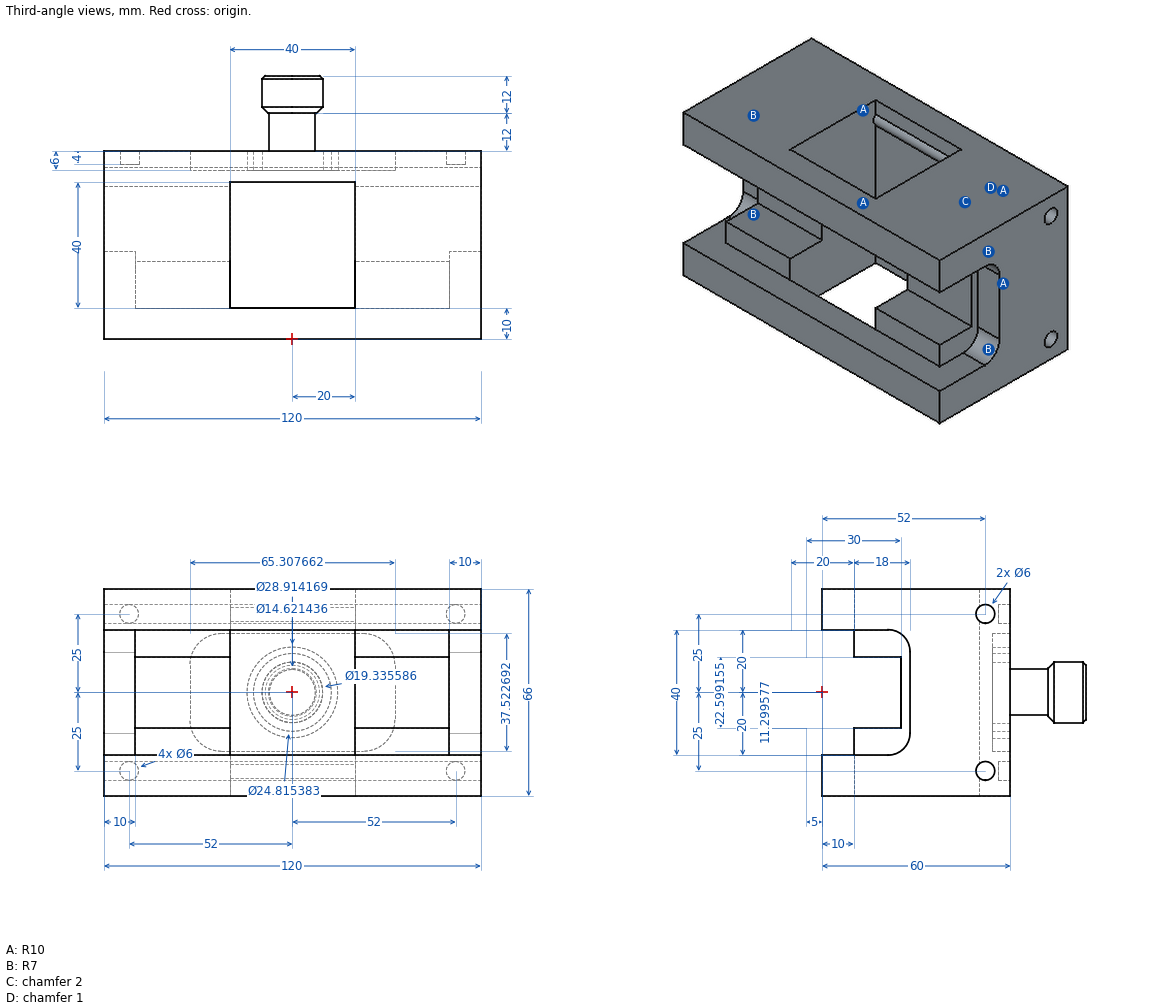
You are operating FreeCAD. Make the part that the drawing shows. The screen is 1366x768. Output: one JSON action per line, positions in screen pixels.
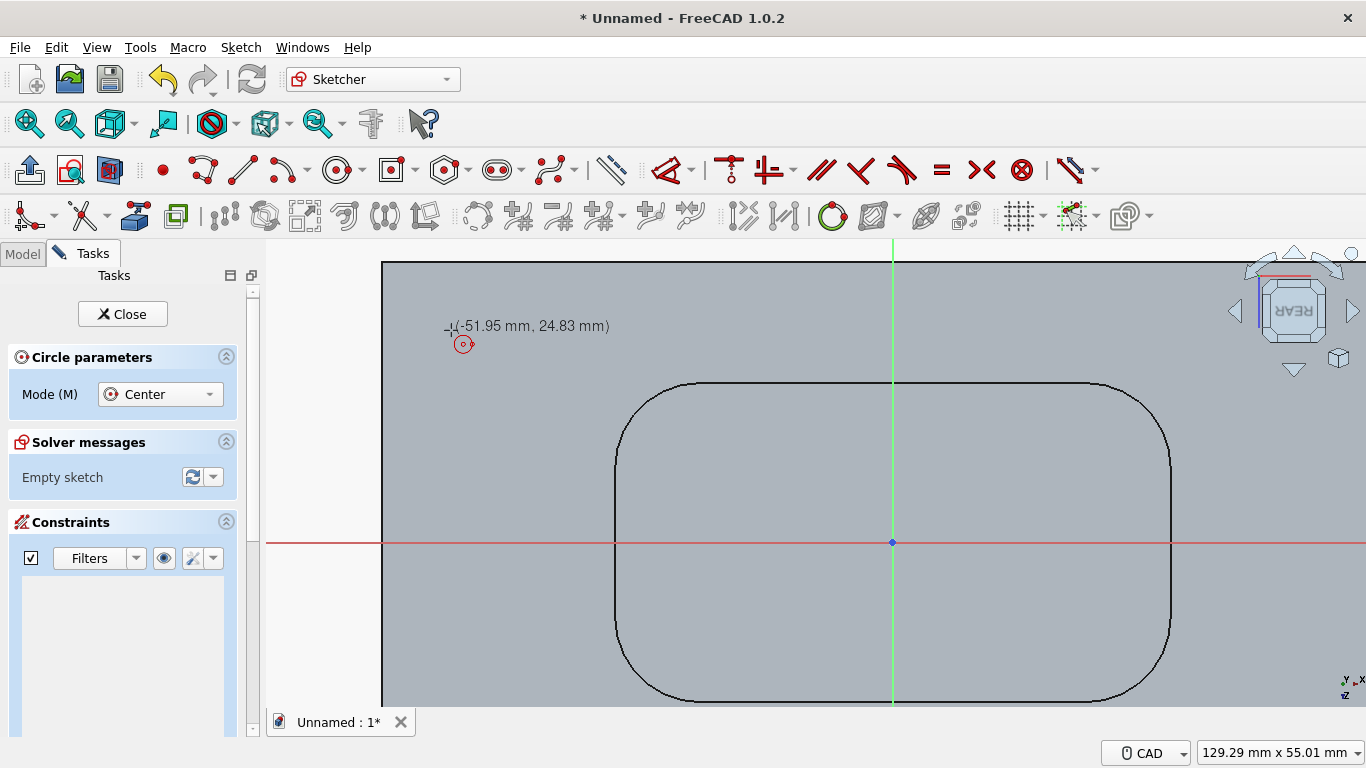
{"action": "left_click", "coordinate": [450, 330]}
{"action": "mouse_move", "coordinate": [469, 312]}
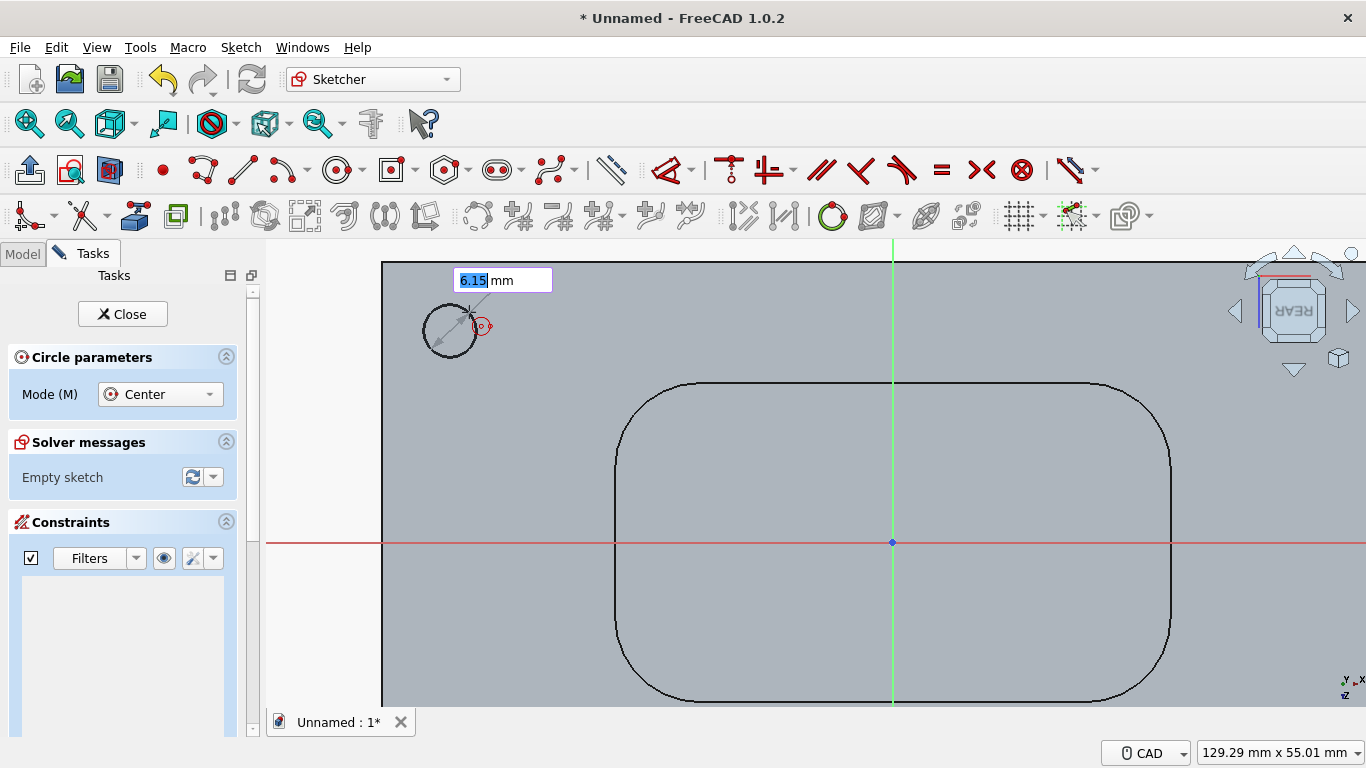
{"action": "type", "text": "6"}
{"action": "key", "text": "Return"}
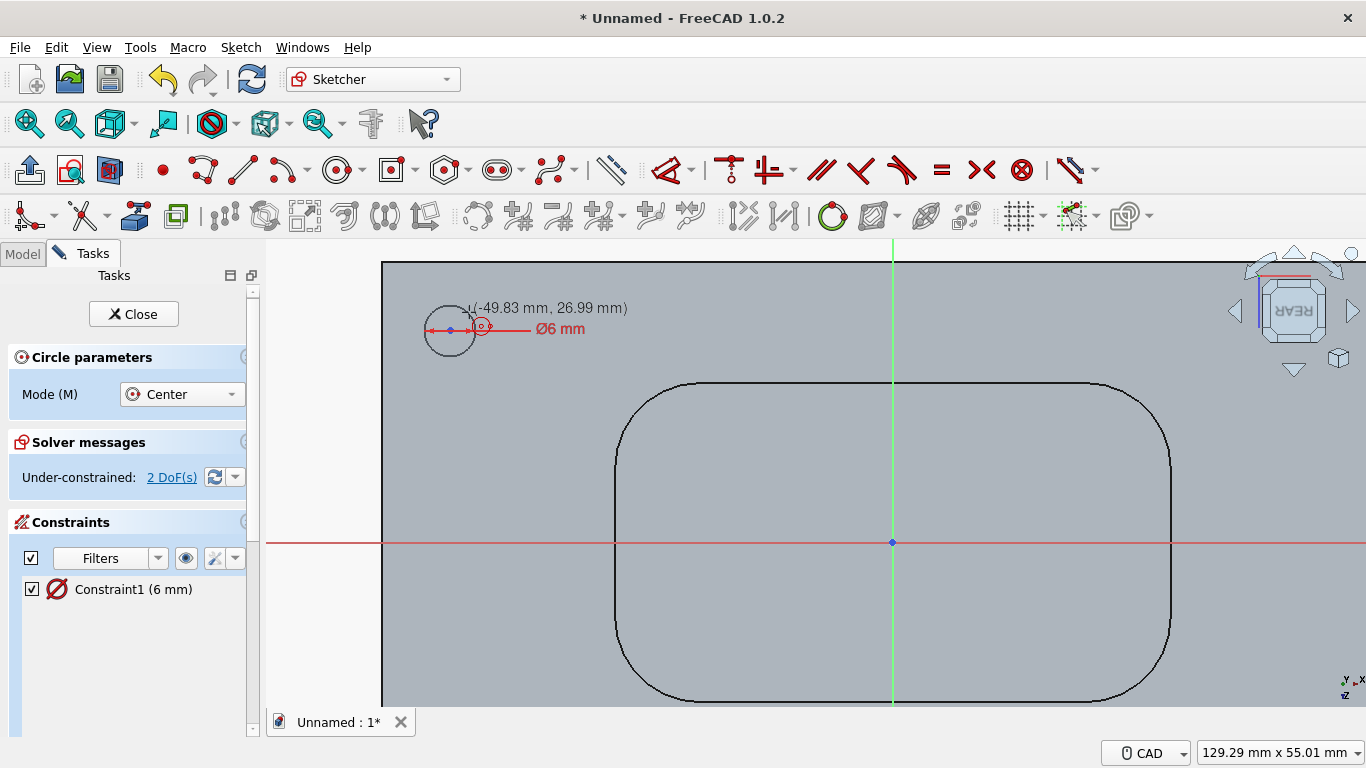
{"action": "scroll", "coordinate": [452, 331], "scroll_direction": "down", "scroll_amount": 2}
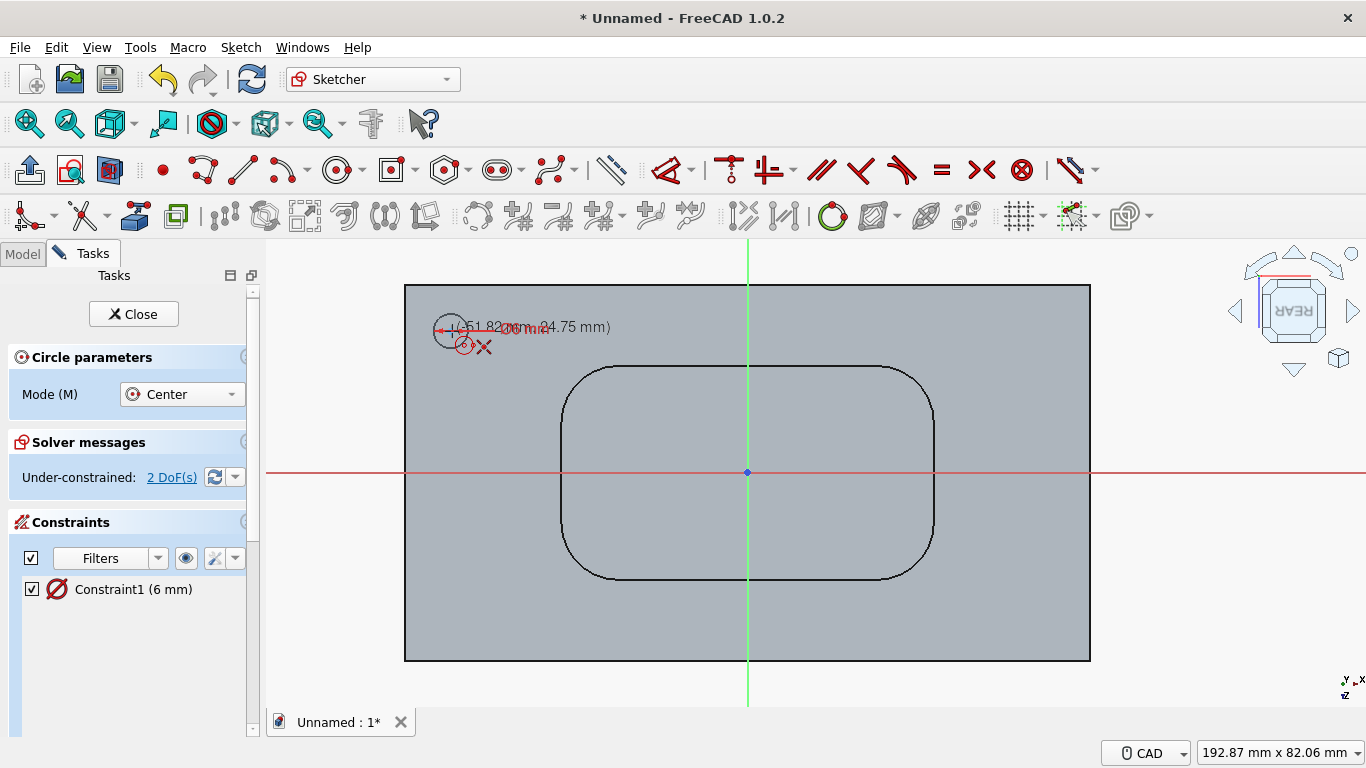
{"action": "scroll", "coordinate": [1044, 330], "scroll_direction": "up", "scroll_amount": 2}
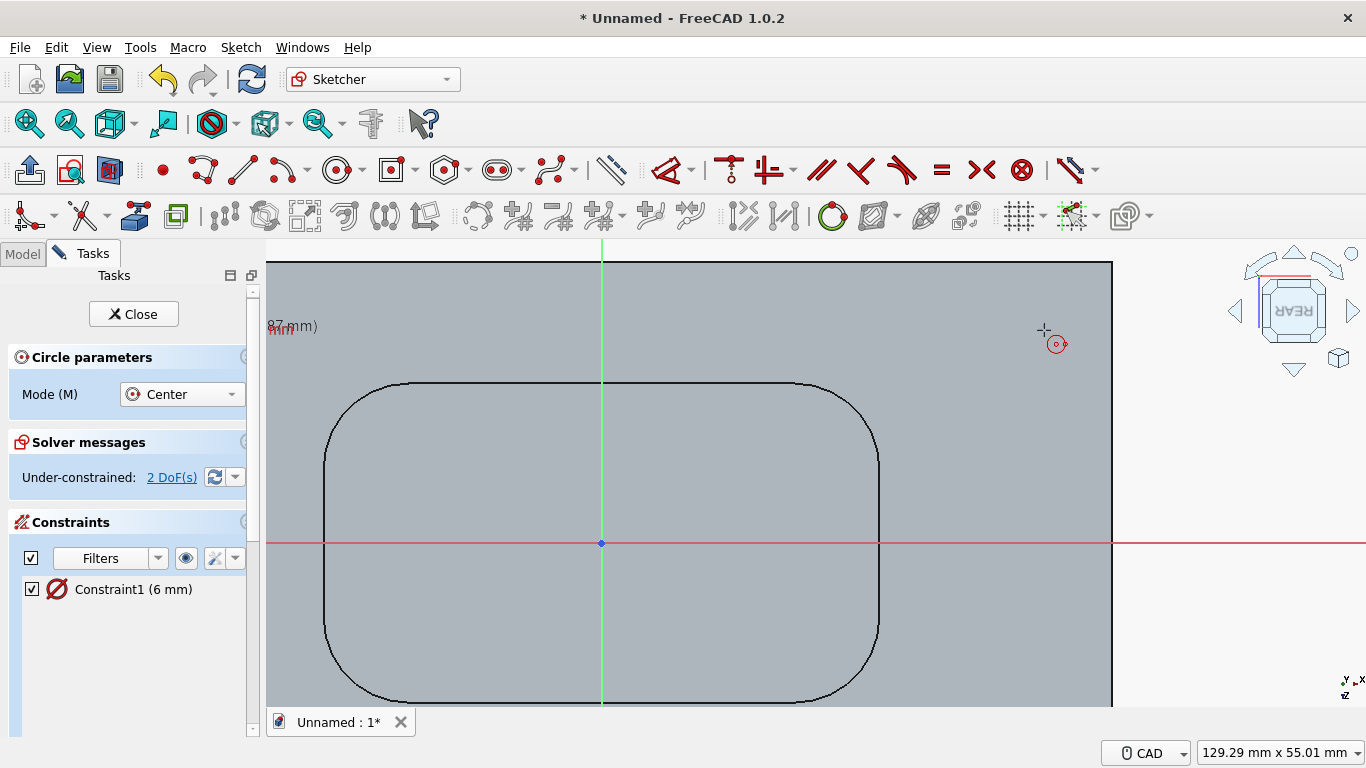
{"action": "left_click", "coordinate": [1044, 330]}
{"action": "mouse_move", "coordinate": [1062, 312]}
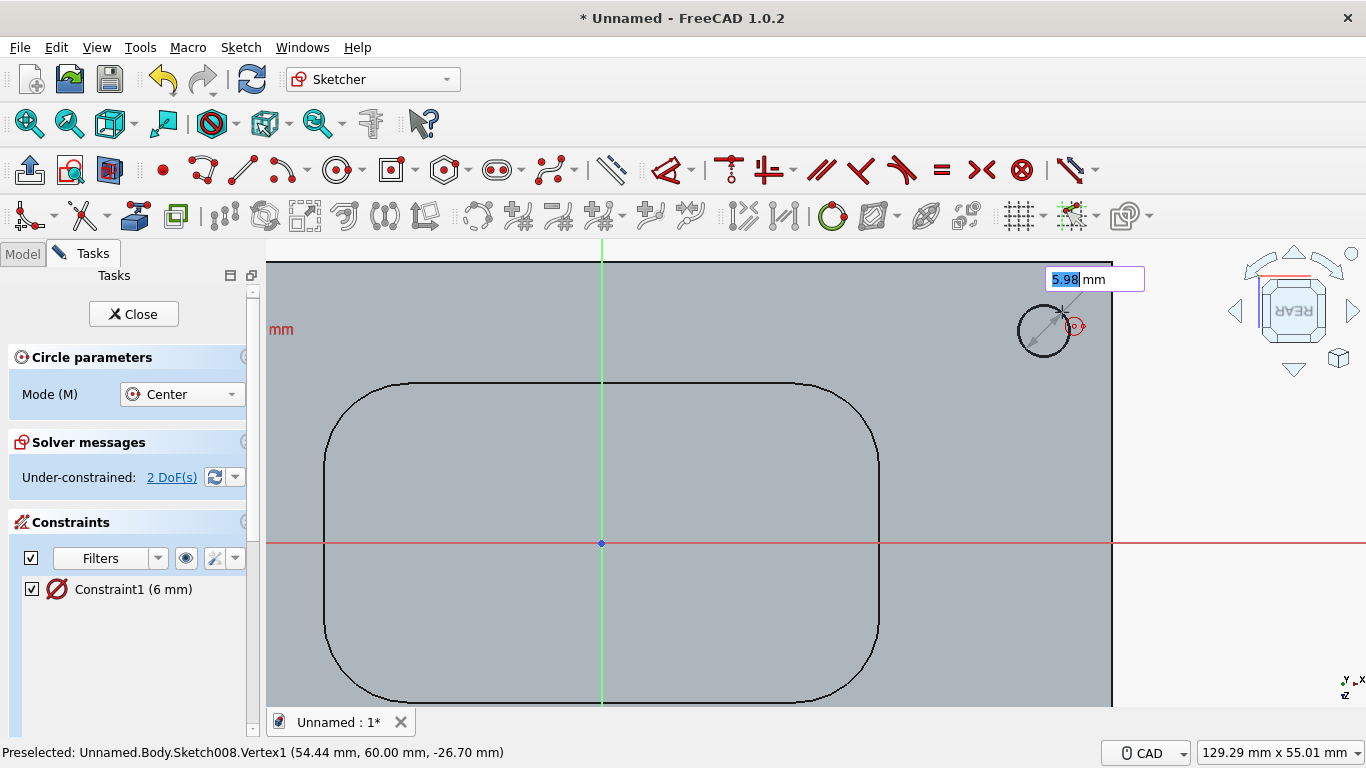
{"action": "type", "text": "6"}
{"action": "key", "text": "Return"}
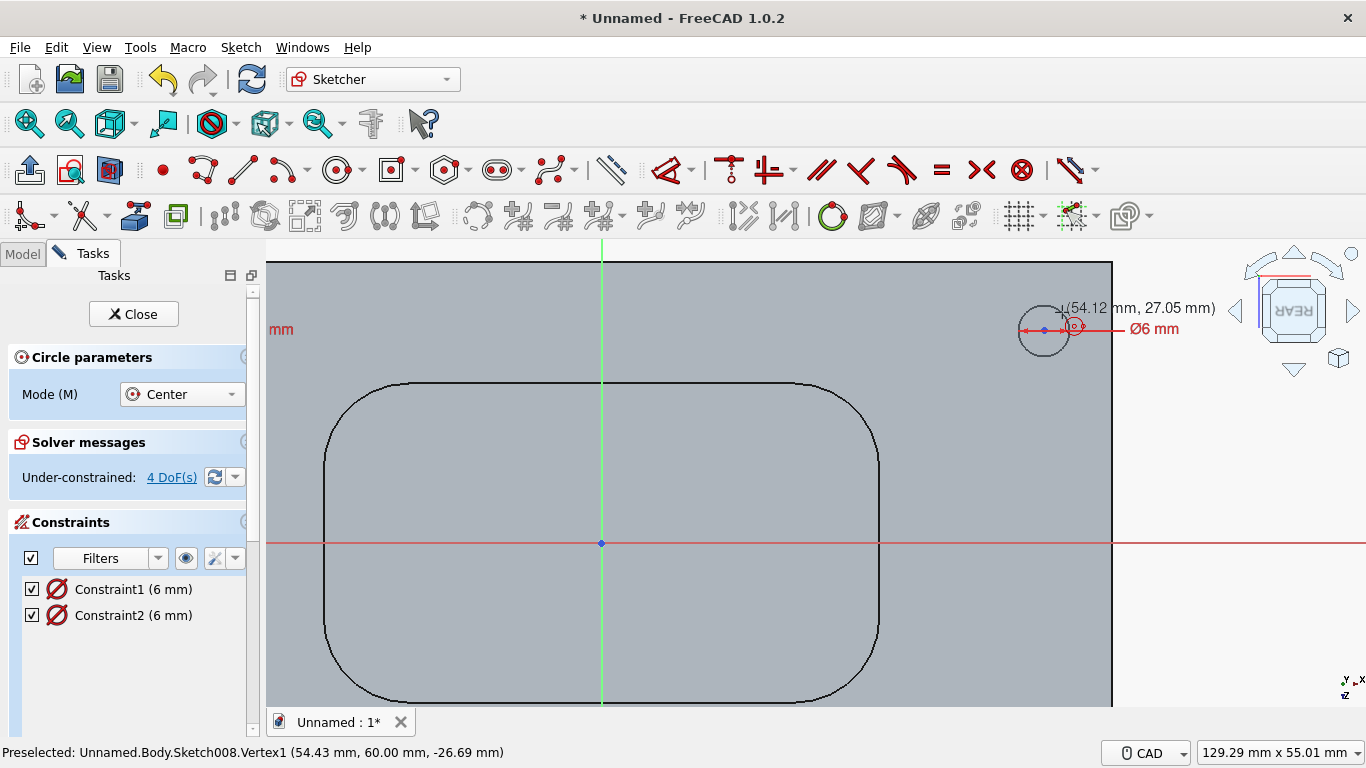
{"action": "scroll", "coordinate": [1044, 330], "scroll_direction": "down", "scroll_amount": 2}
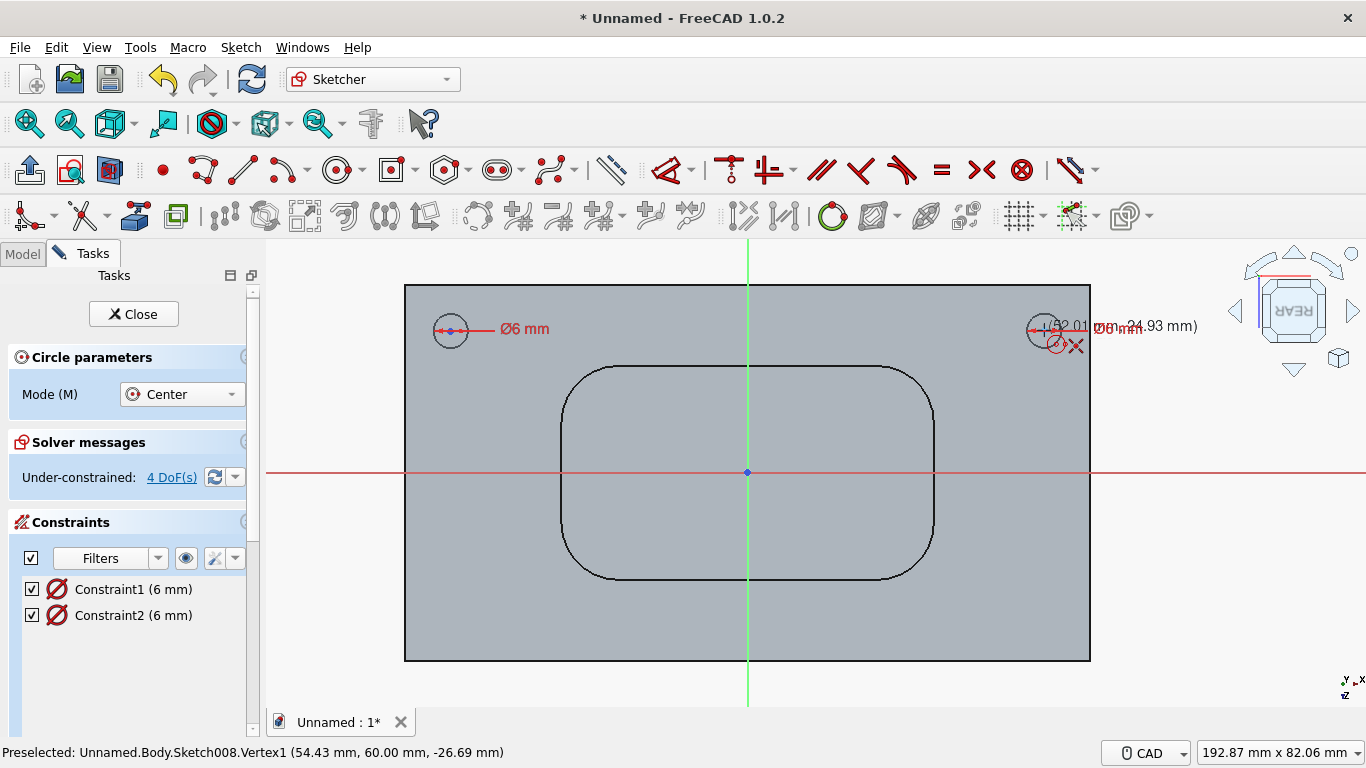
{"action": "scroll", "coordinate": [451, 616], "scroll_direction": "up", "scroll_amount": 2}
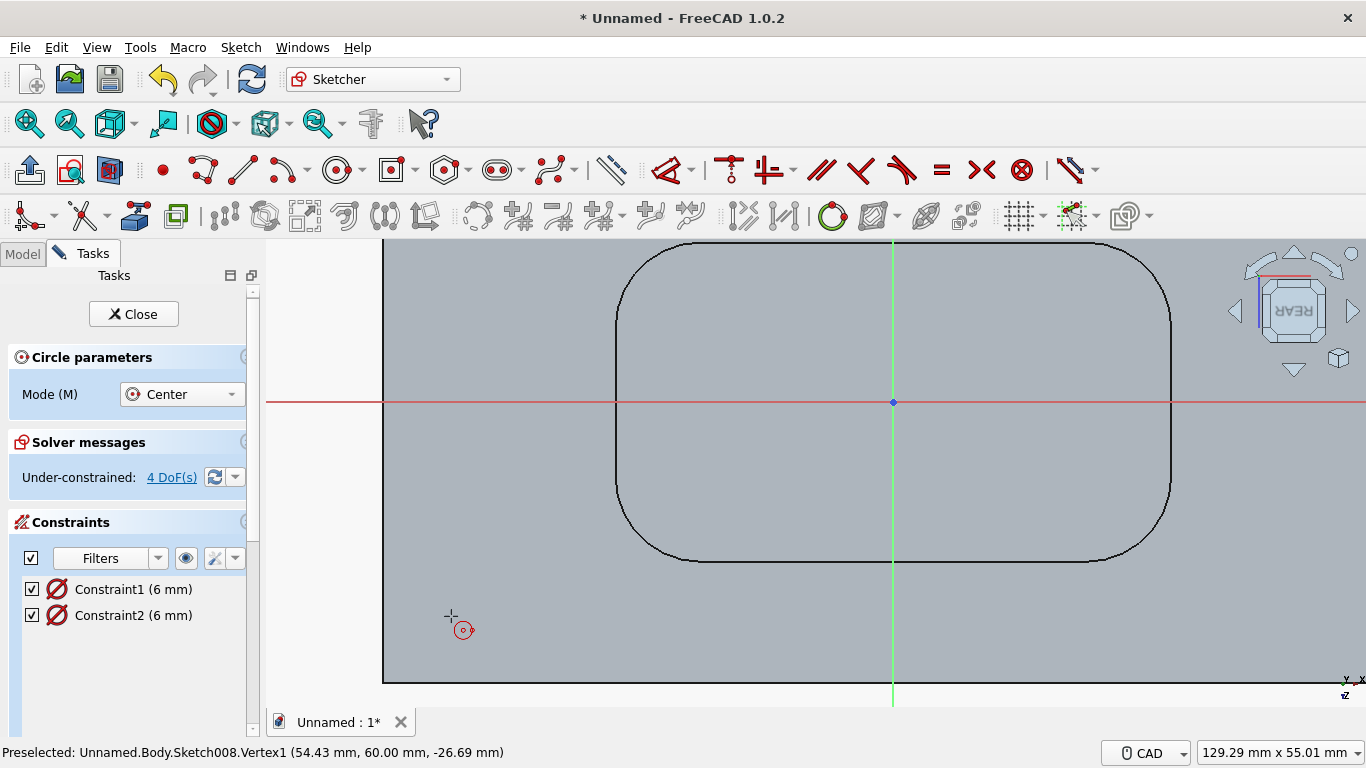
{"action": "left_click", "coordinate": [451, 615]}
{"action": "mouse_move", "coordinate": [469, 597]}